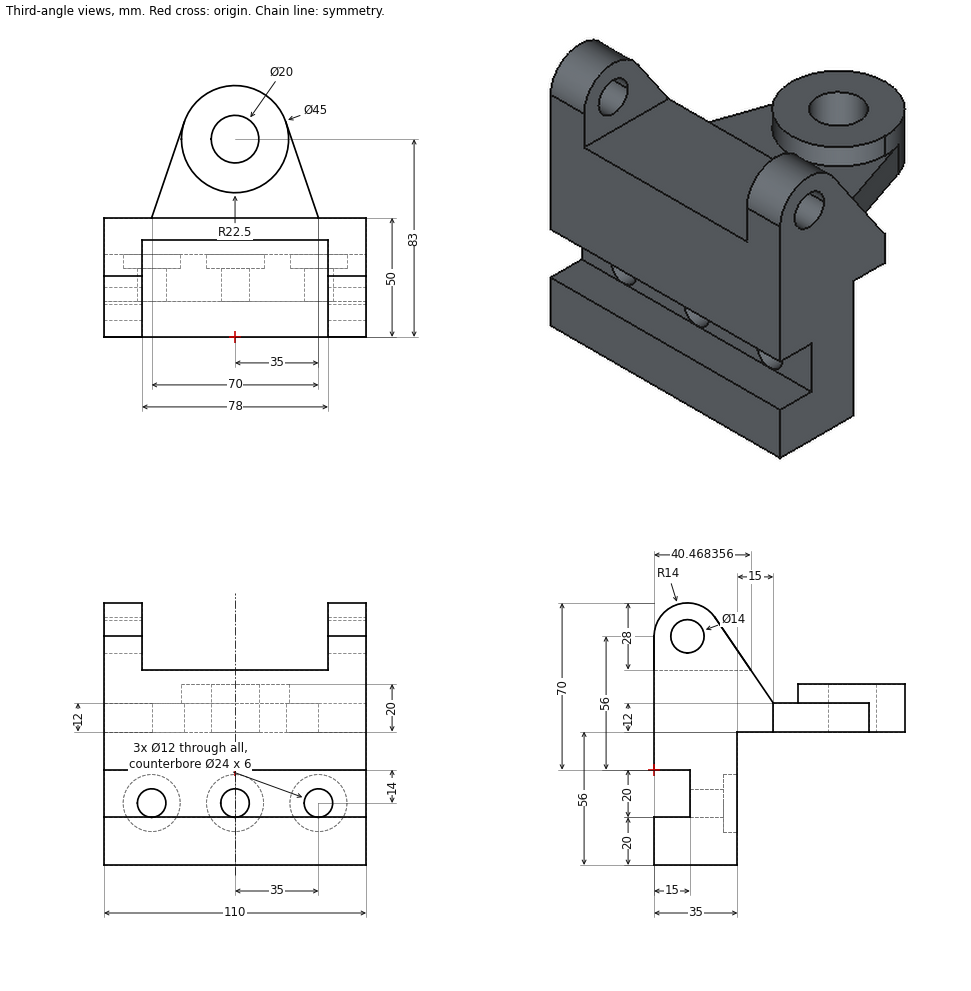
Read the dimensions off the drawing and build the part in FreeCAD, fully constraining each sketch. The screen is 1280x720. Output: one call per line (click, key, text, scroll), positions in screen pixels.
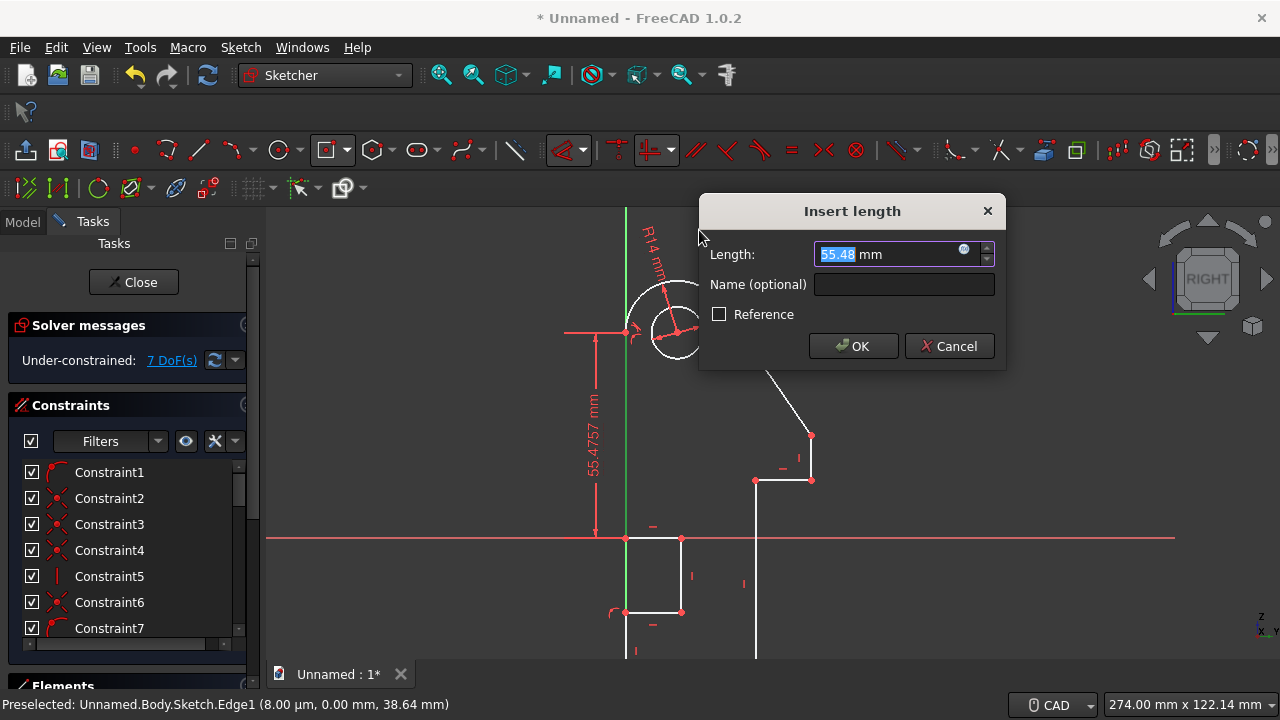
text(56)
key(Return)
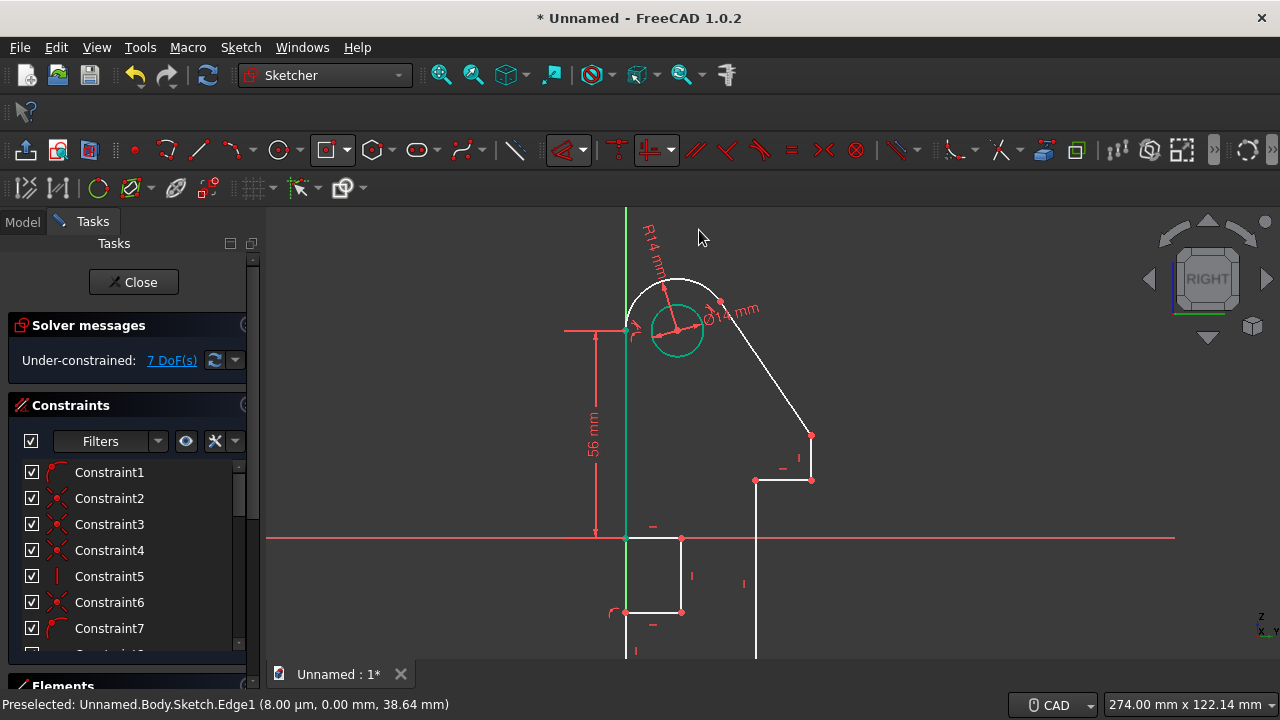
click(642, 538)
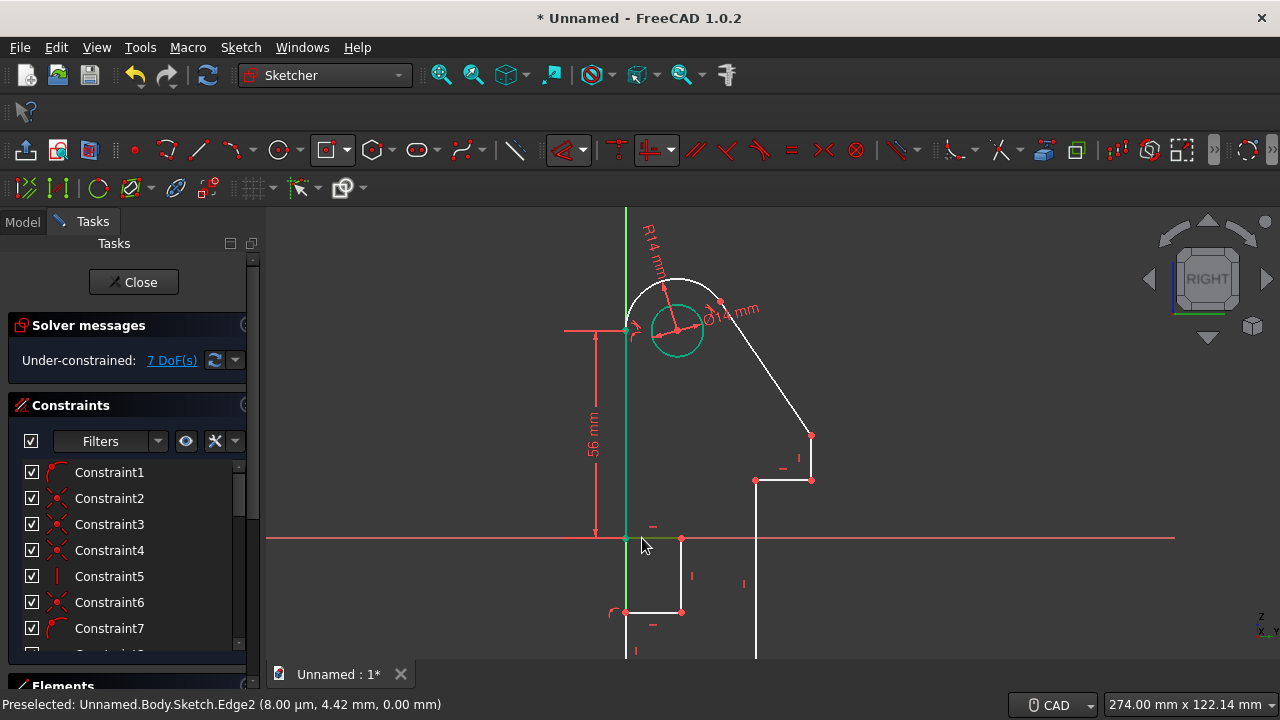
click(586, 150)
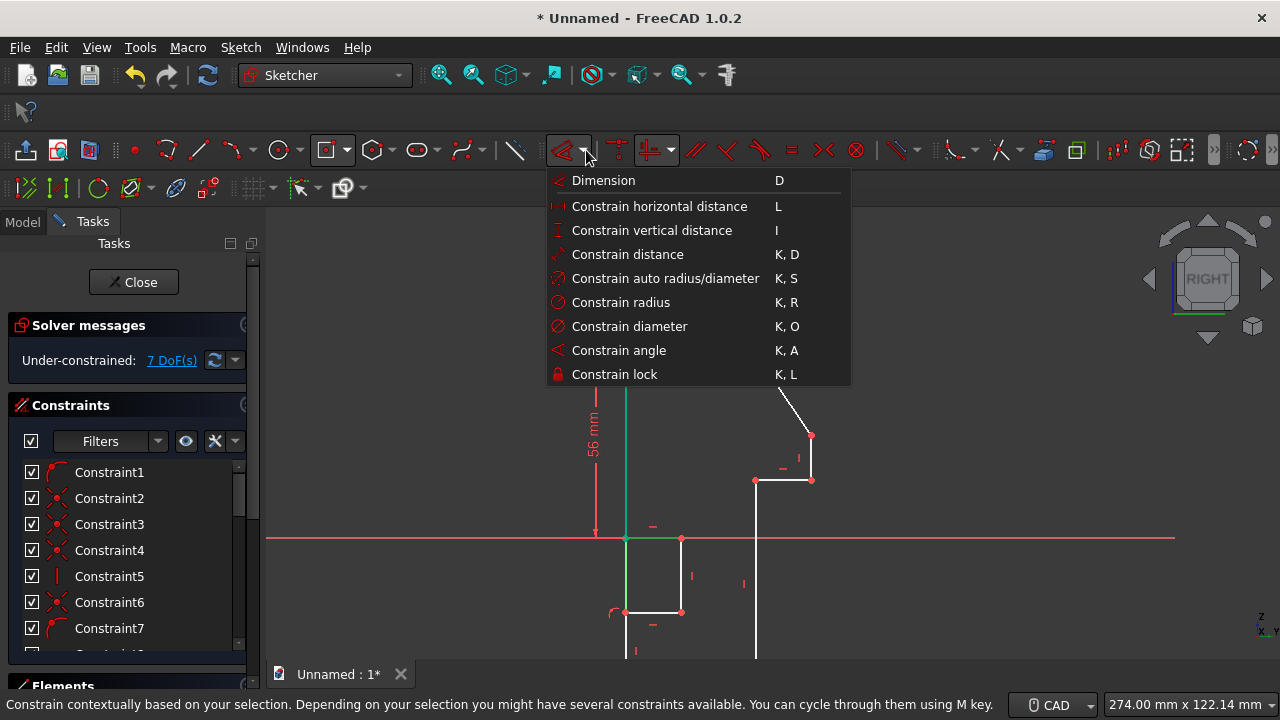
click(699, 206)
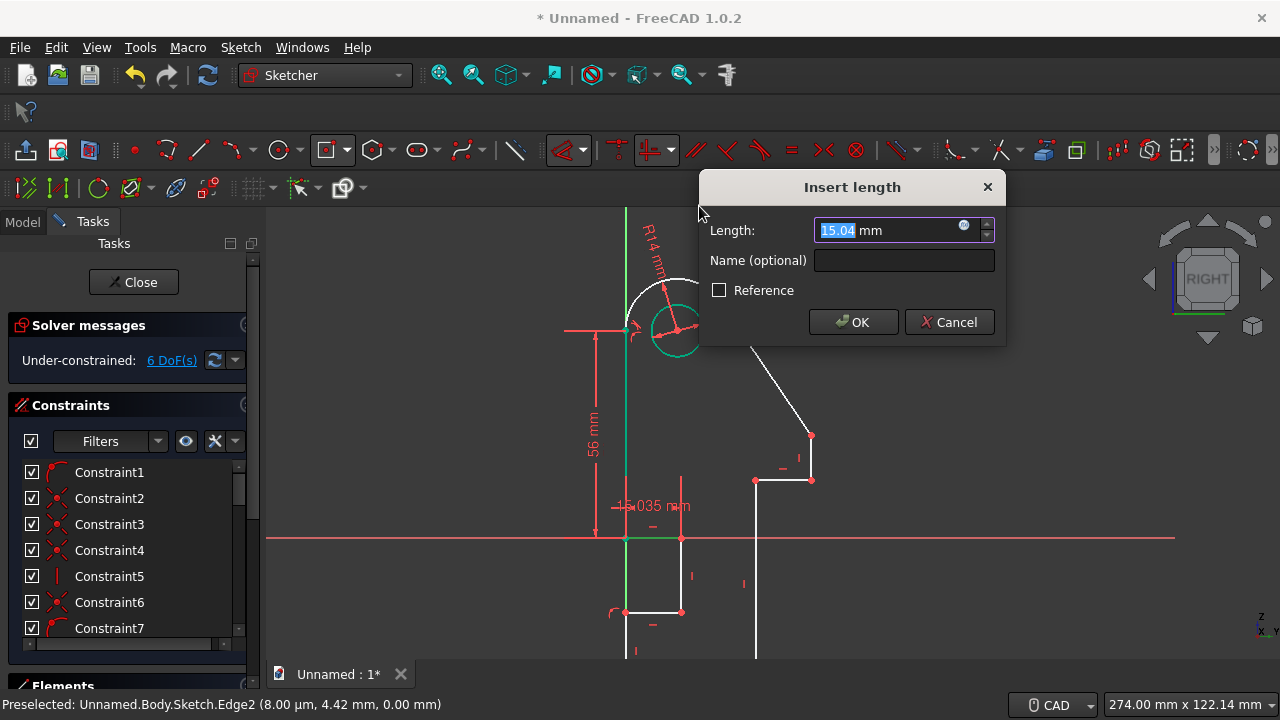
text(15)
key(Return)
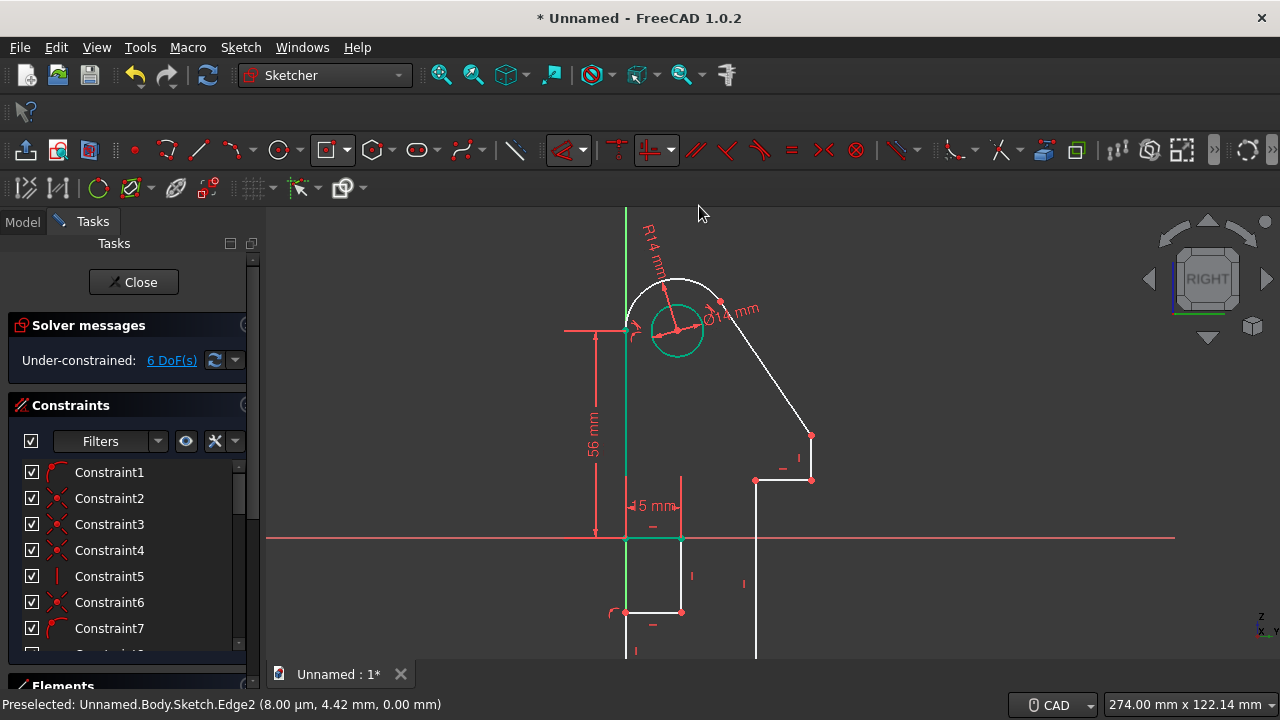
click(681, 560)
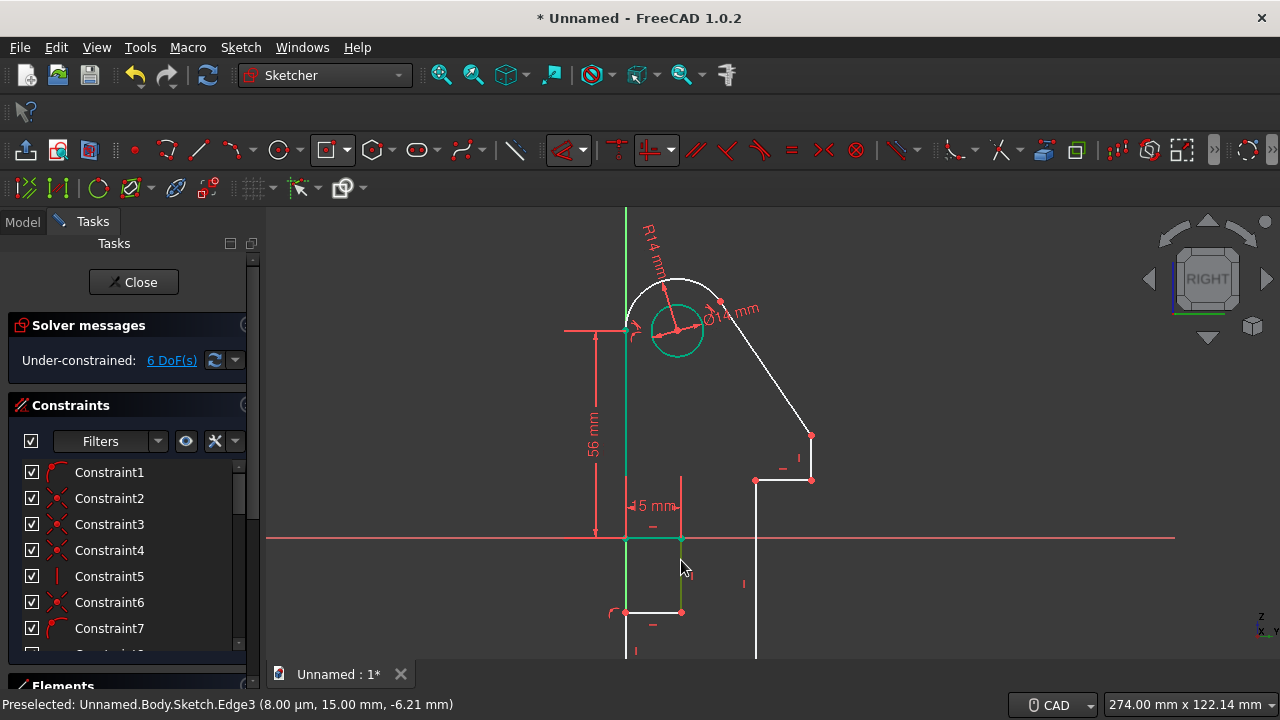
click(586, 150)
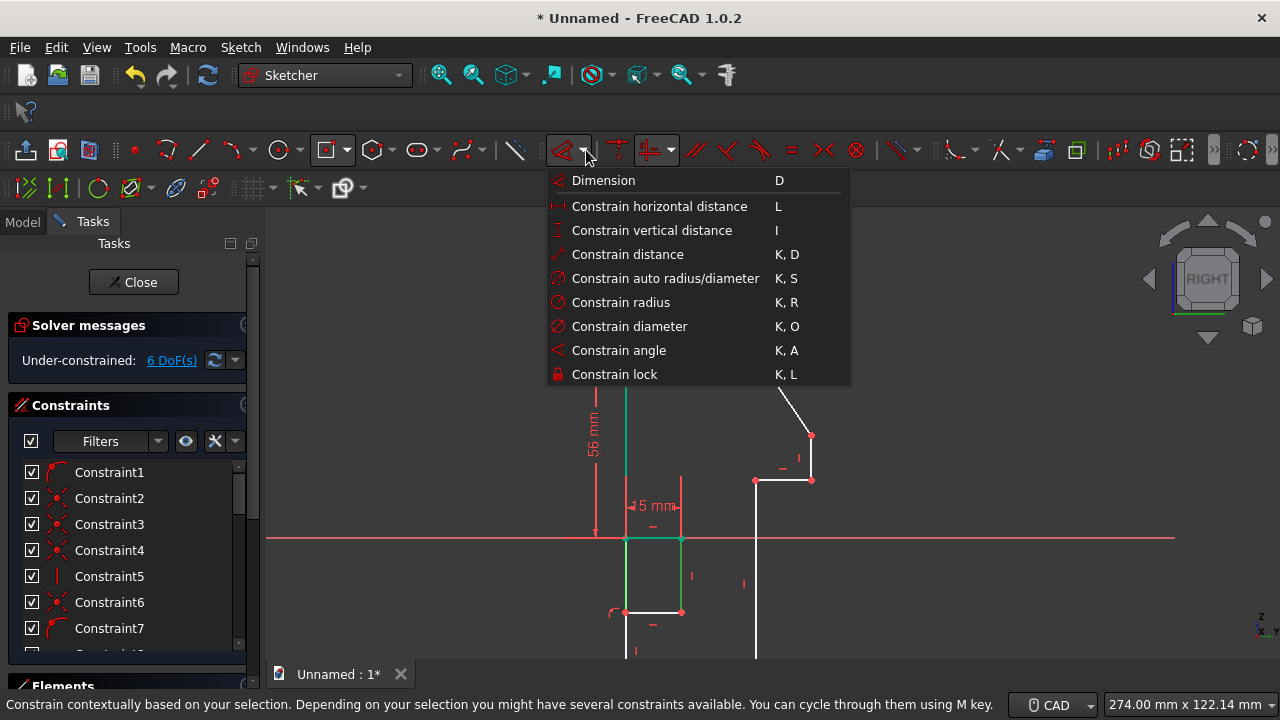
click(699, 230)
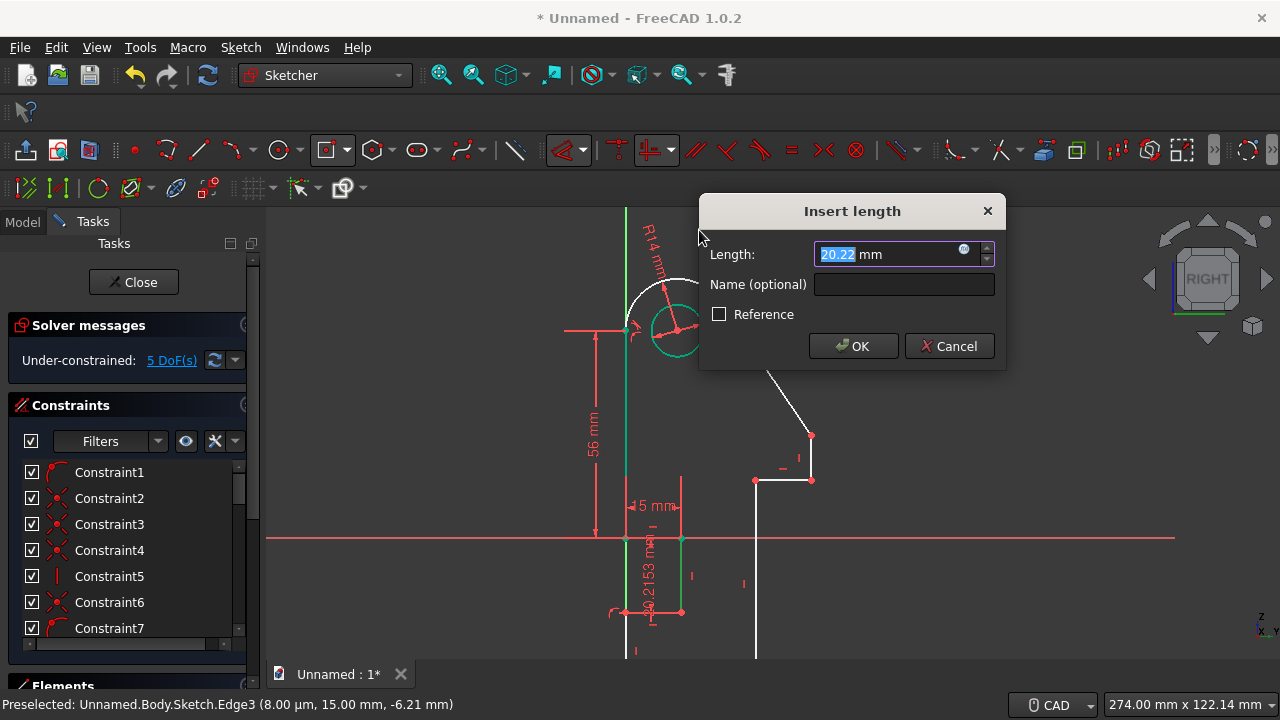
text(20)
key(Return)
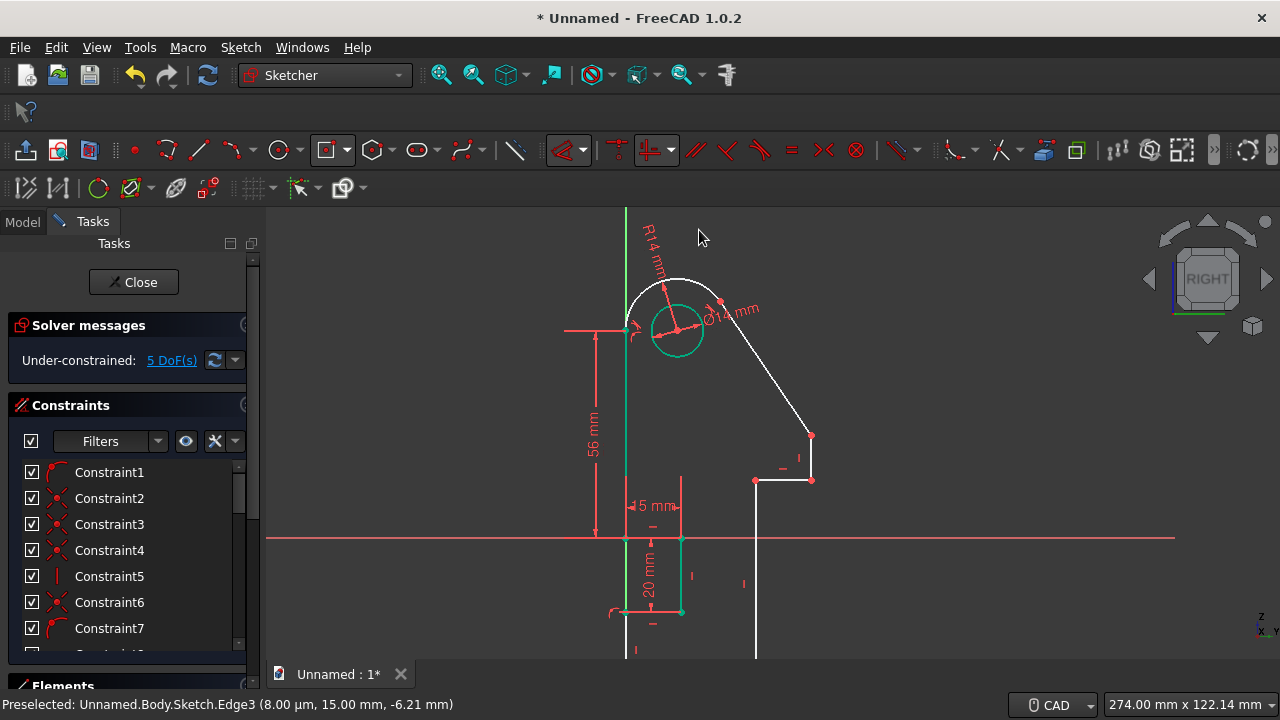
click(626, 627)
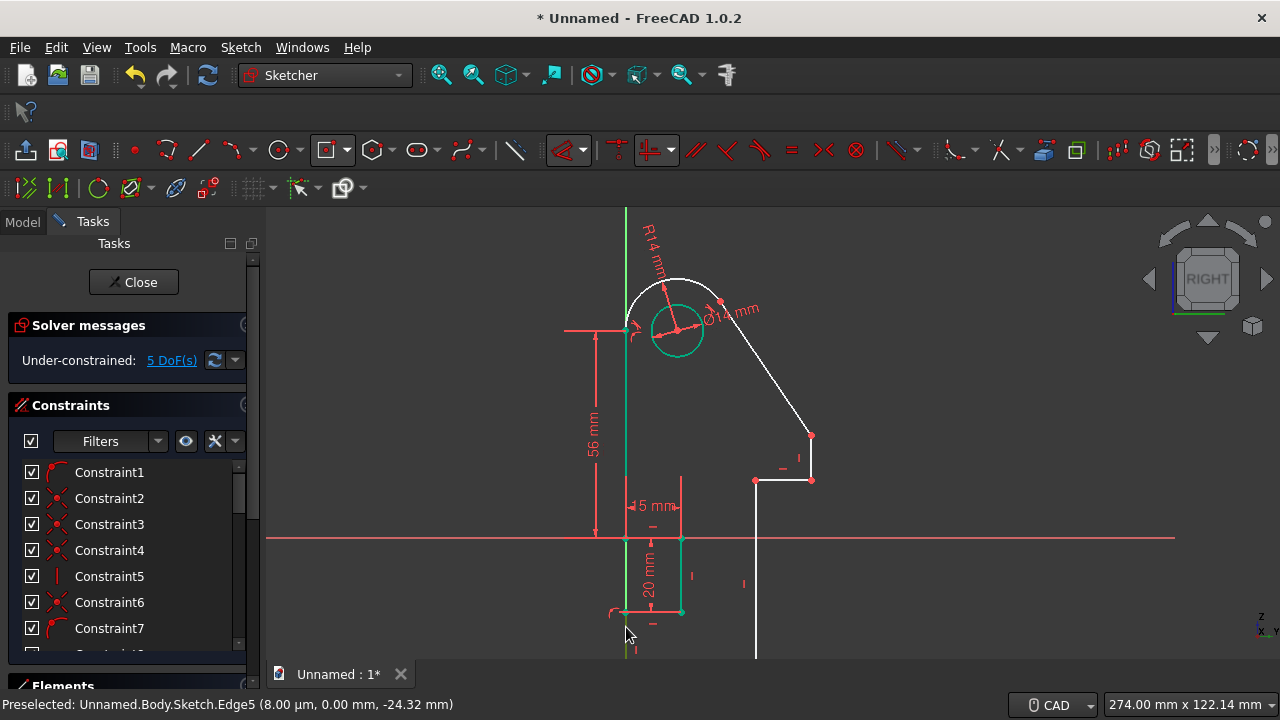
key(i)